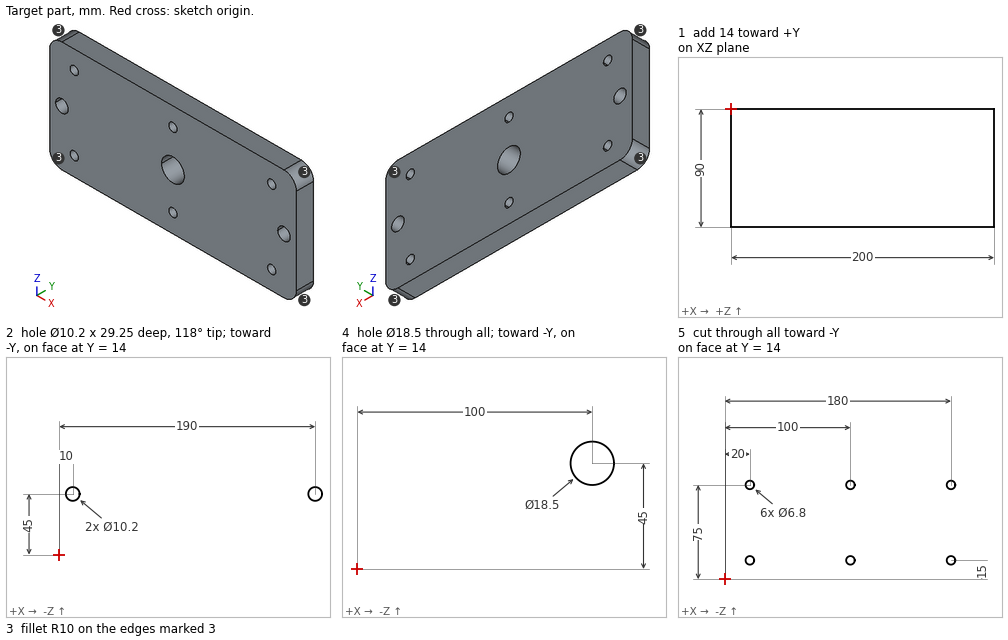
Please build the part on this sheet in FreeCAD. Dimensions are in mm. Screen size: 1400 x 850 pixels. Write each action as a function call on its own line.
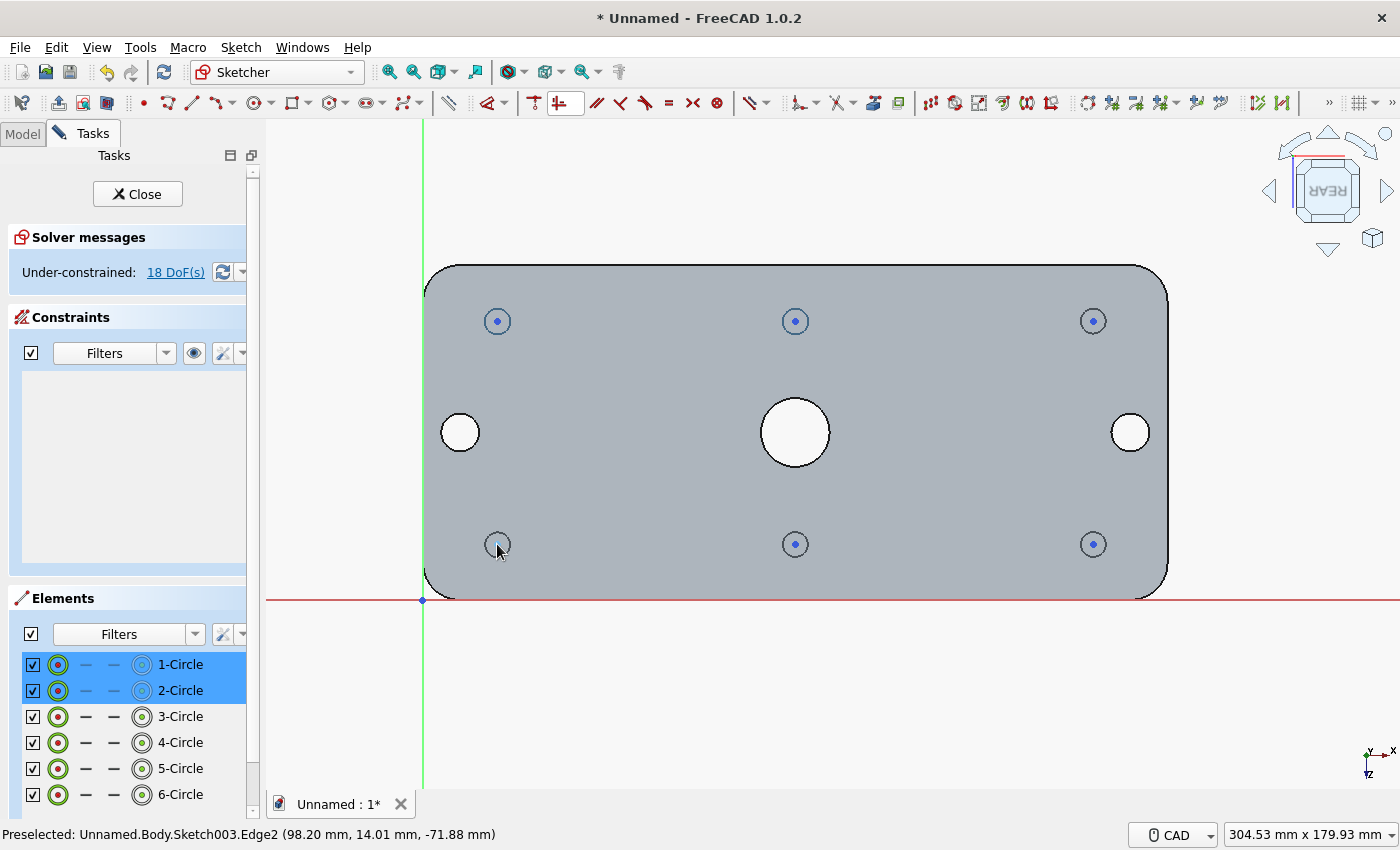
click(1102, 312)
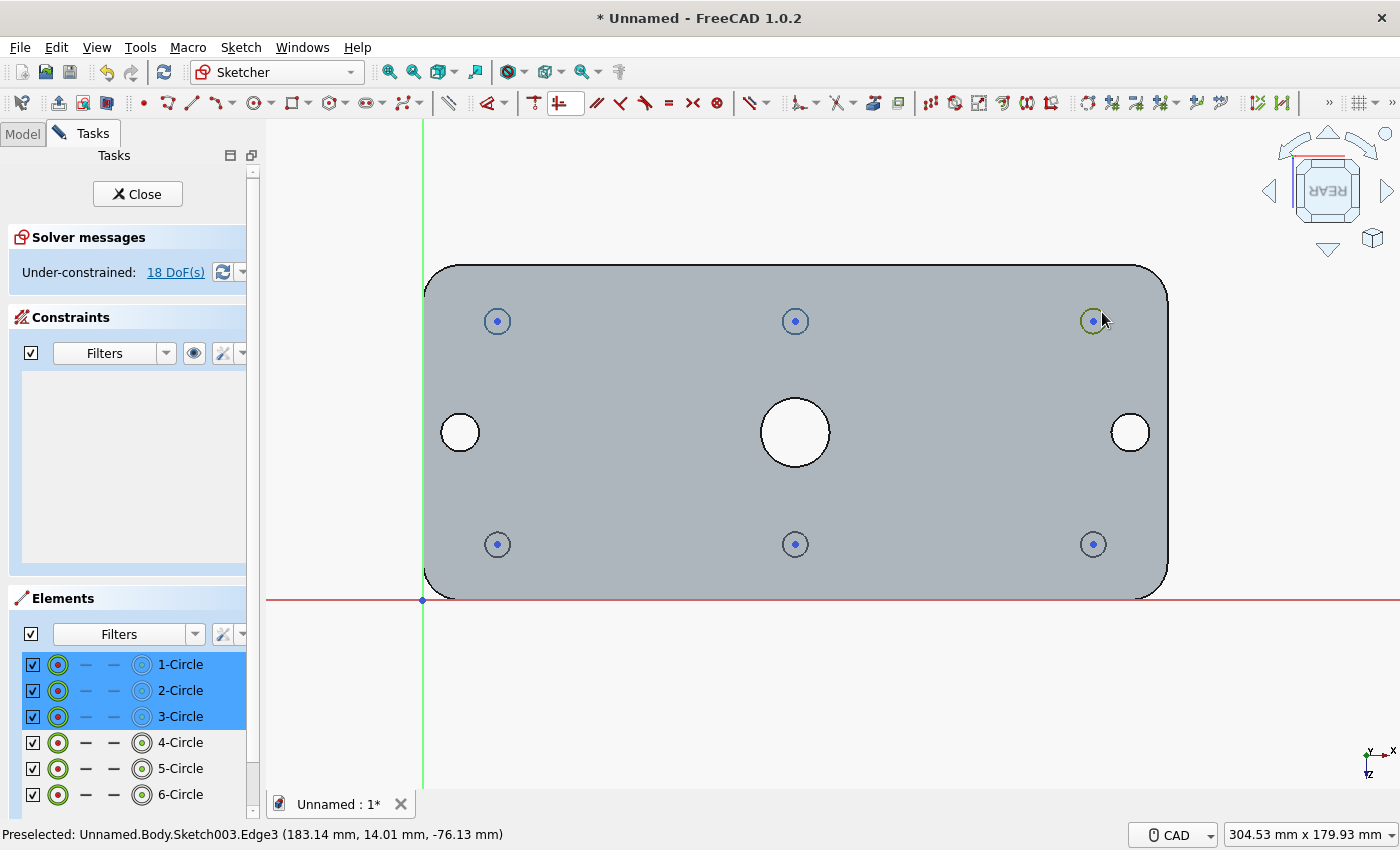
click(1102, 536)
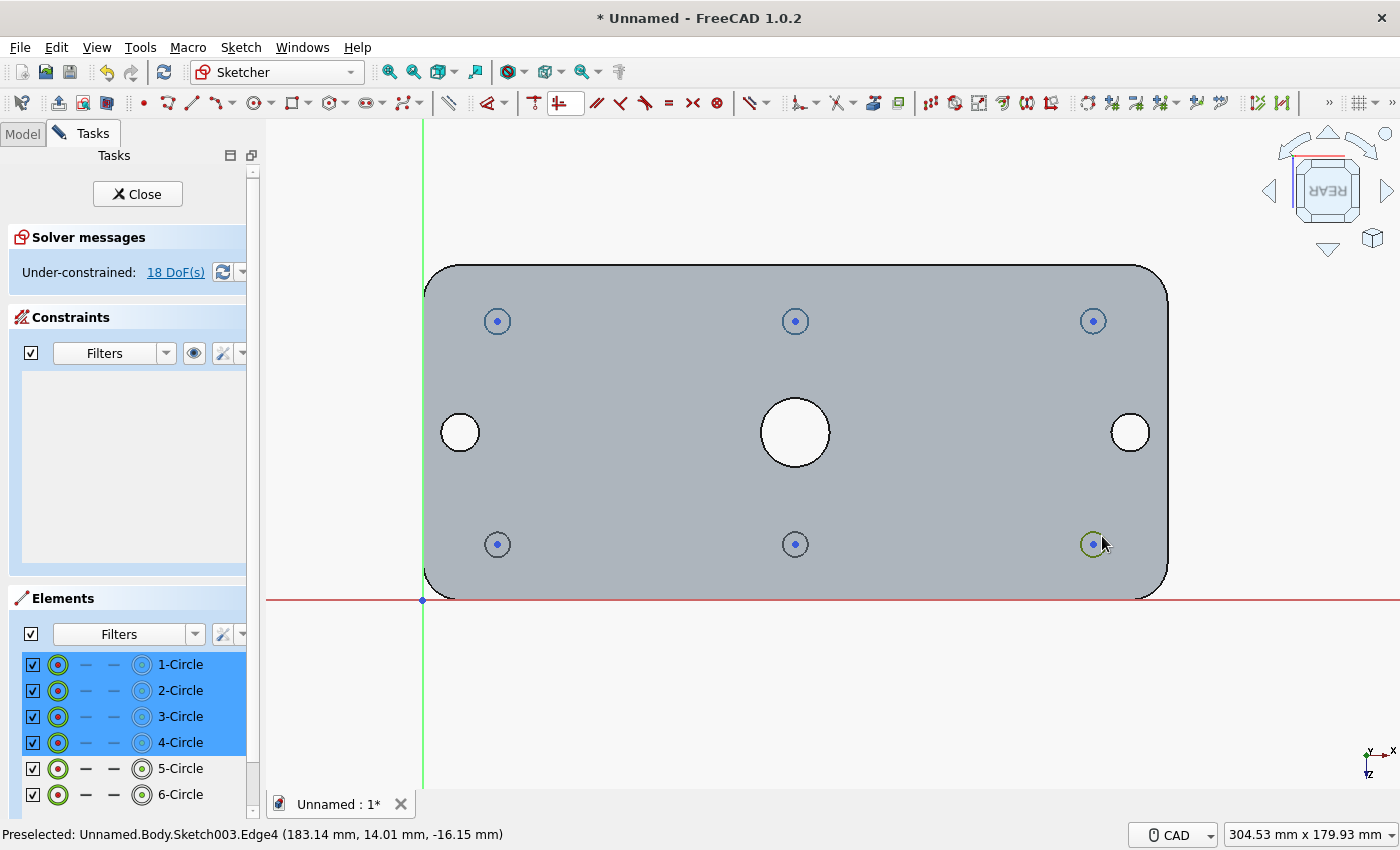
click(804, 536)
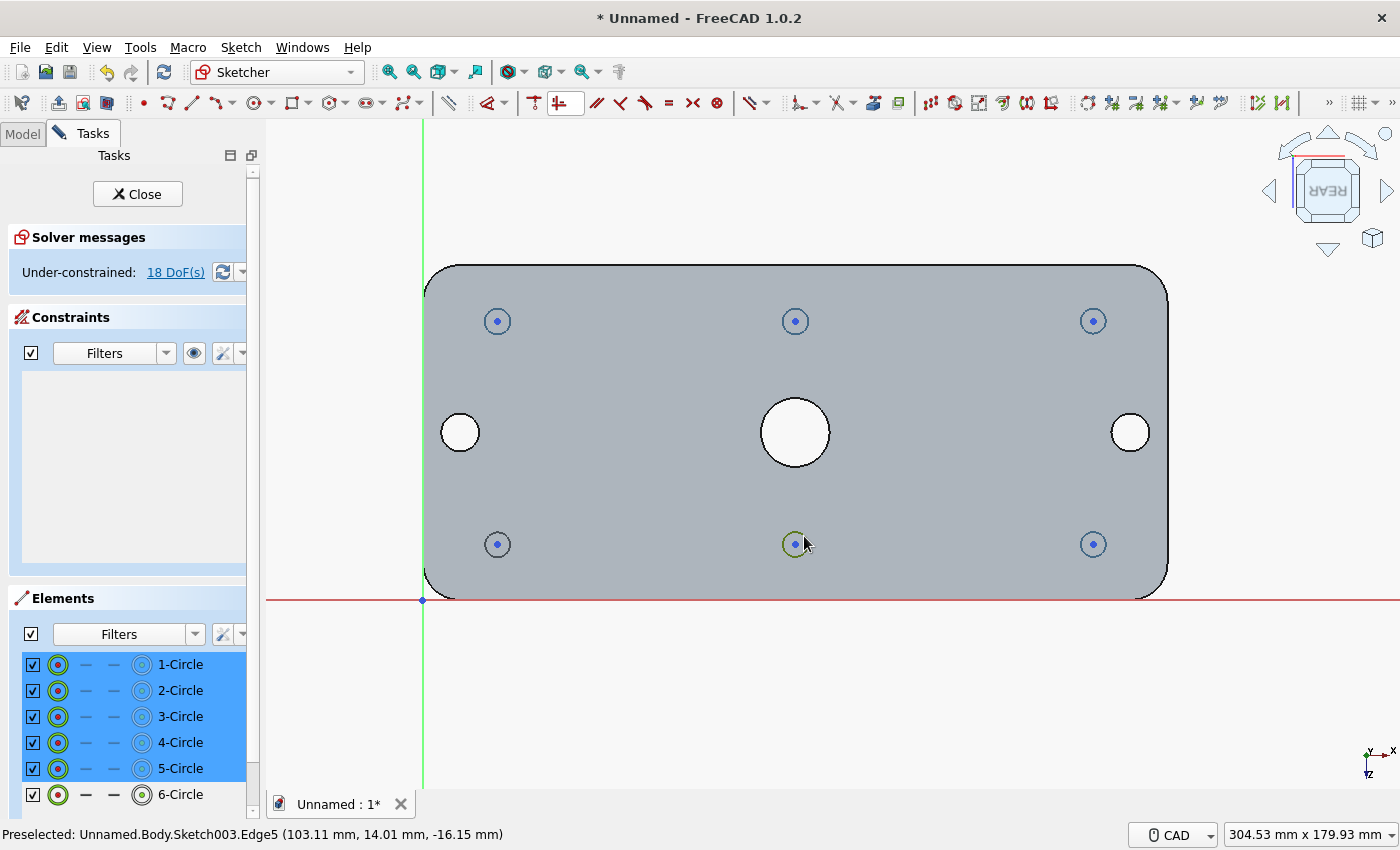
click(506, 536)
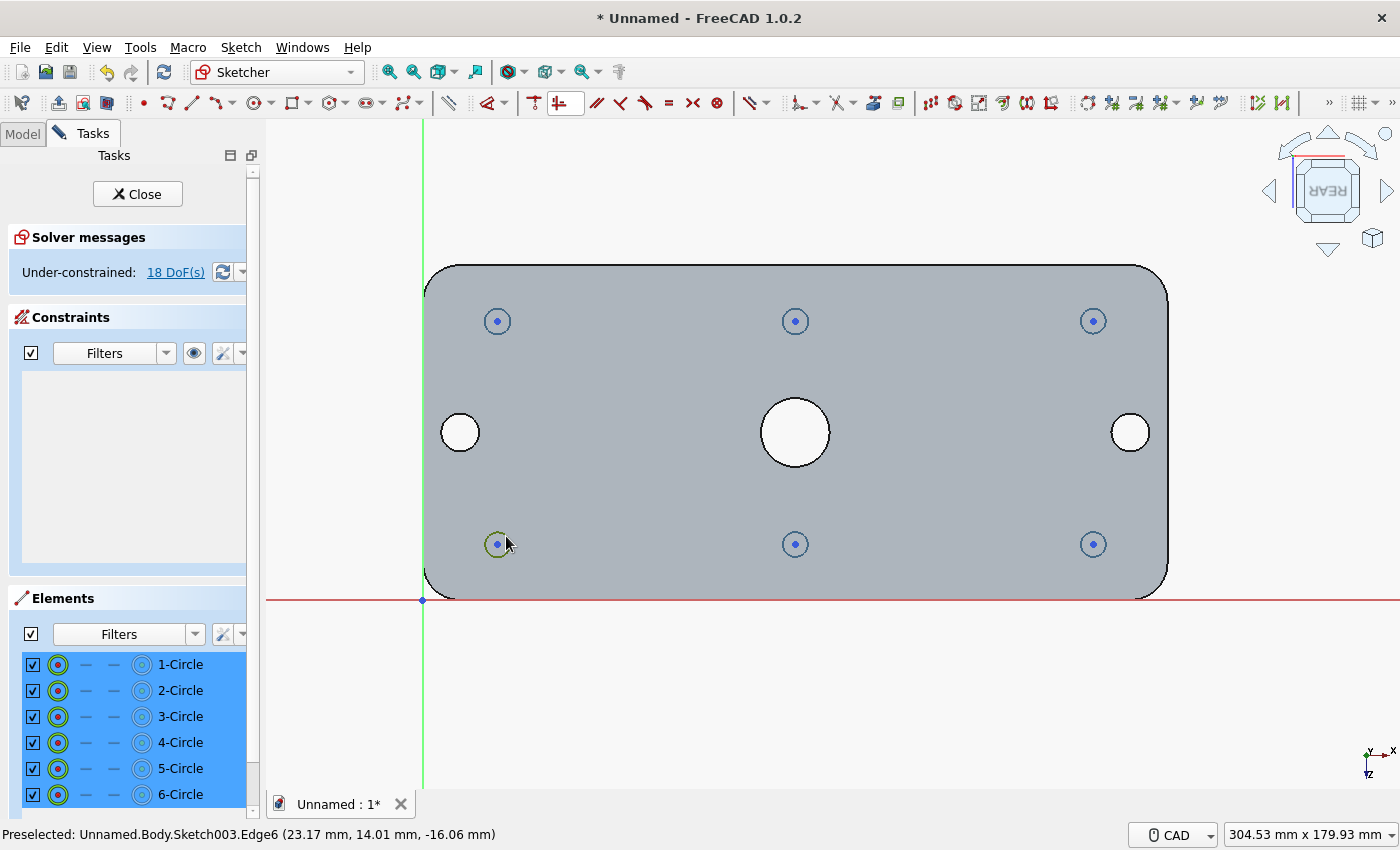
click(670, 104)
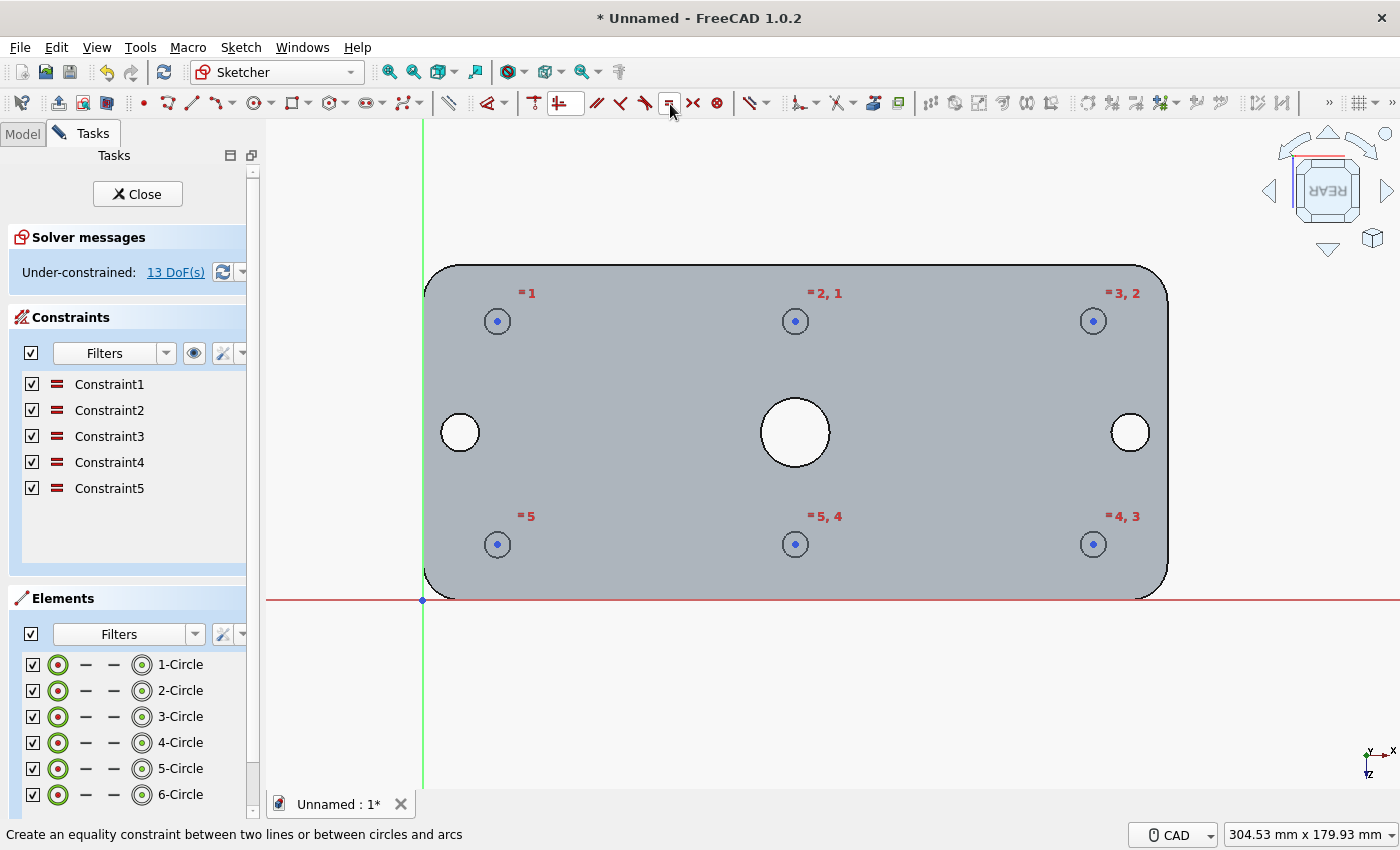
click(497, 322)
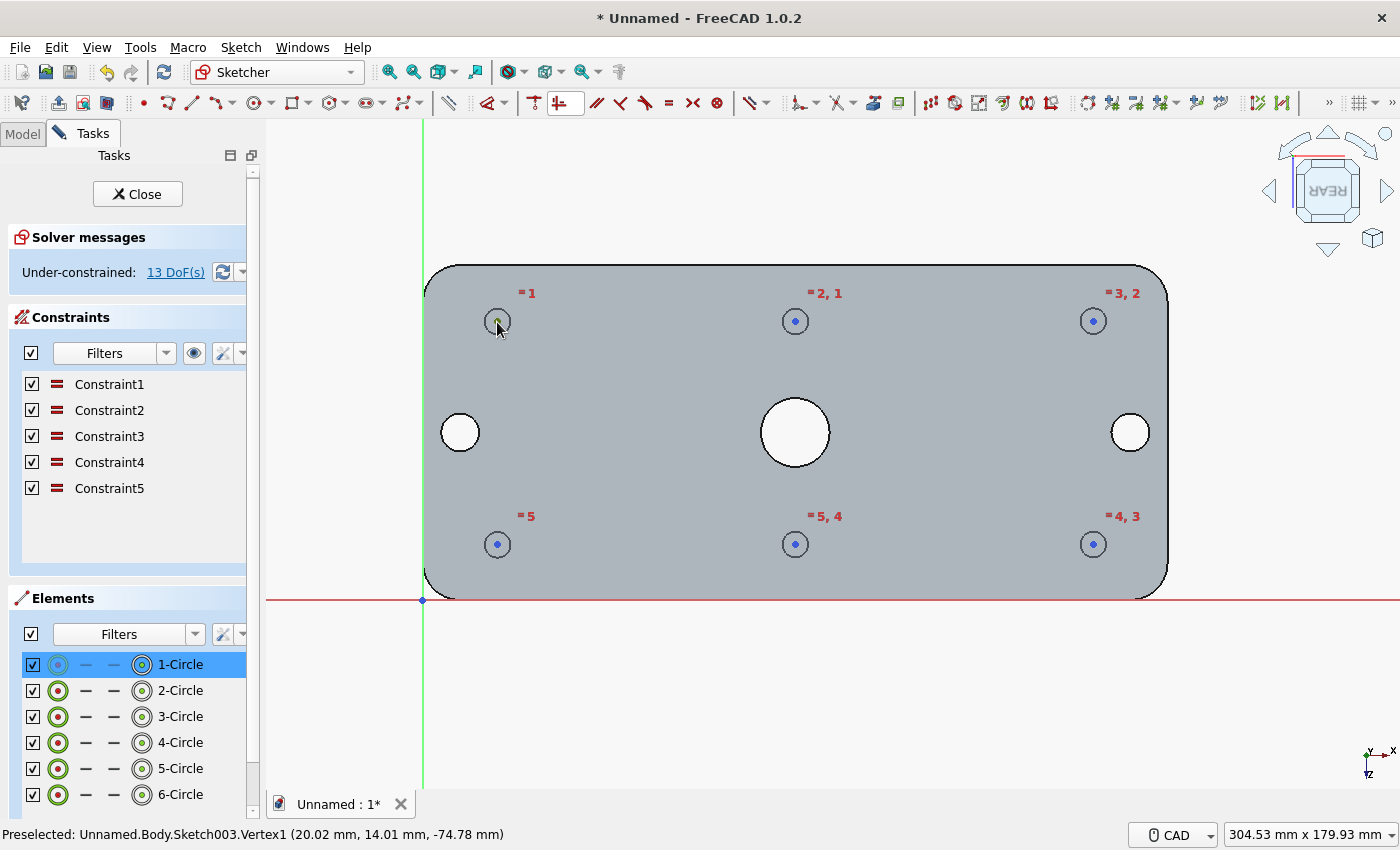
click(795, 322)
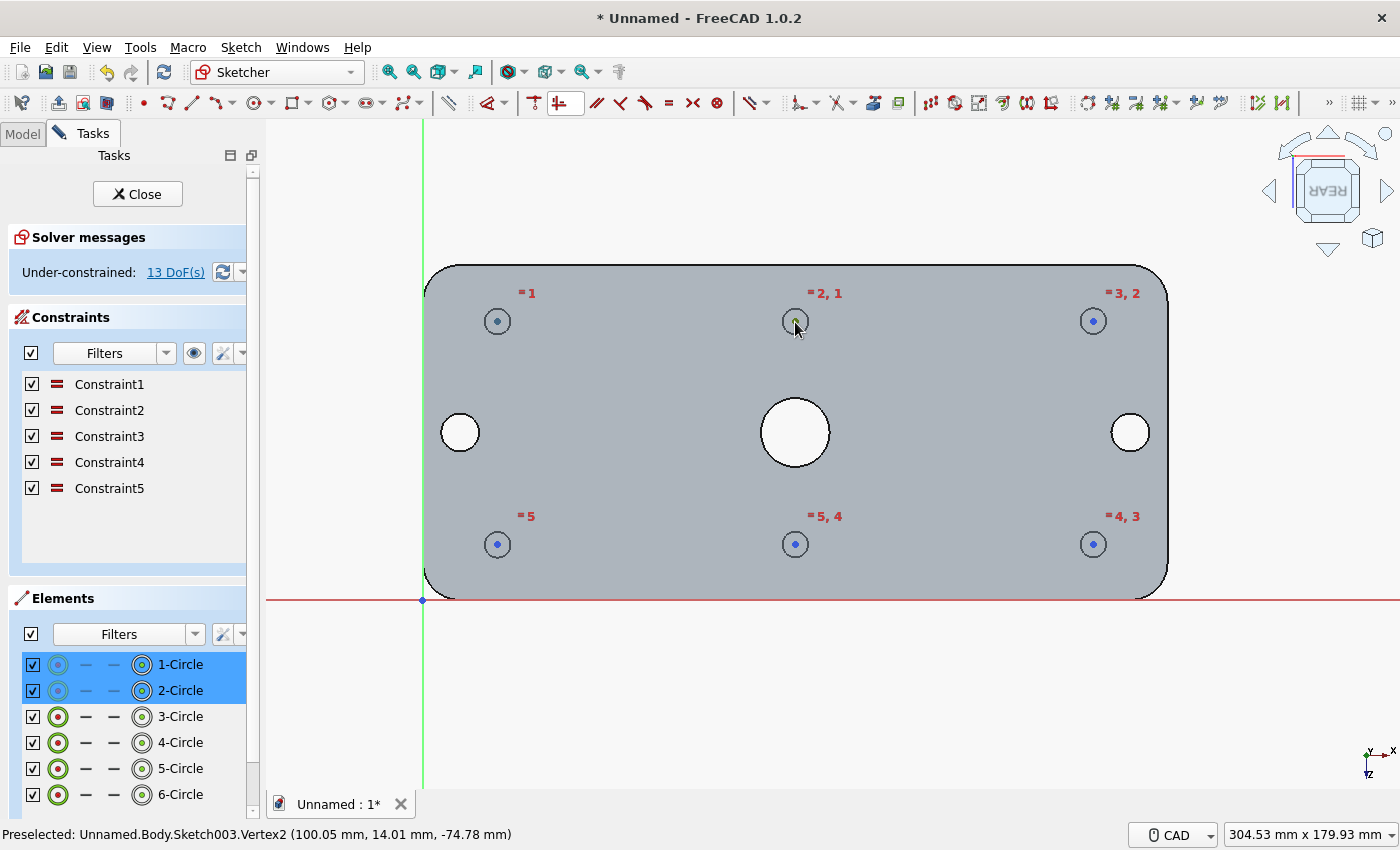
key(h)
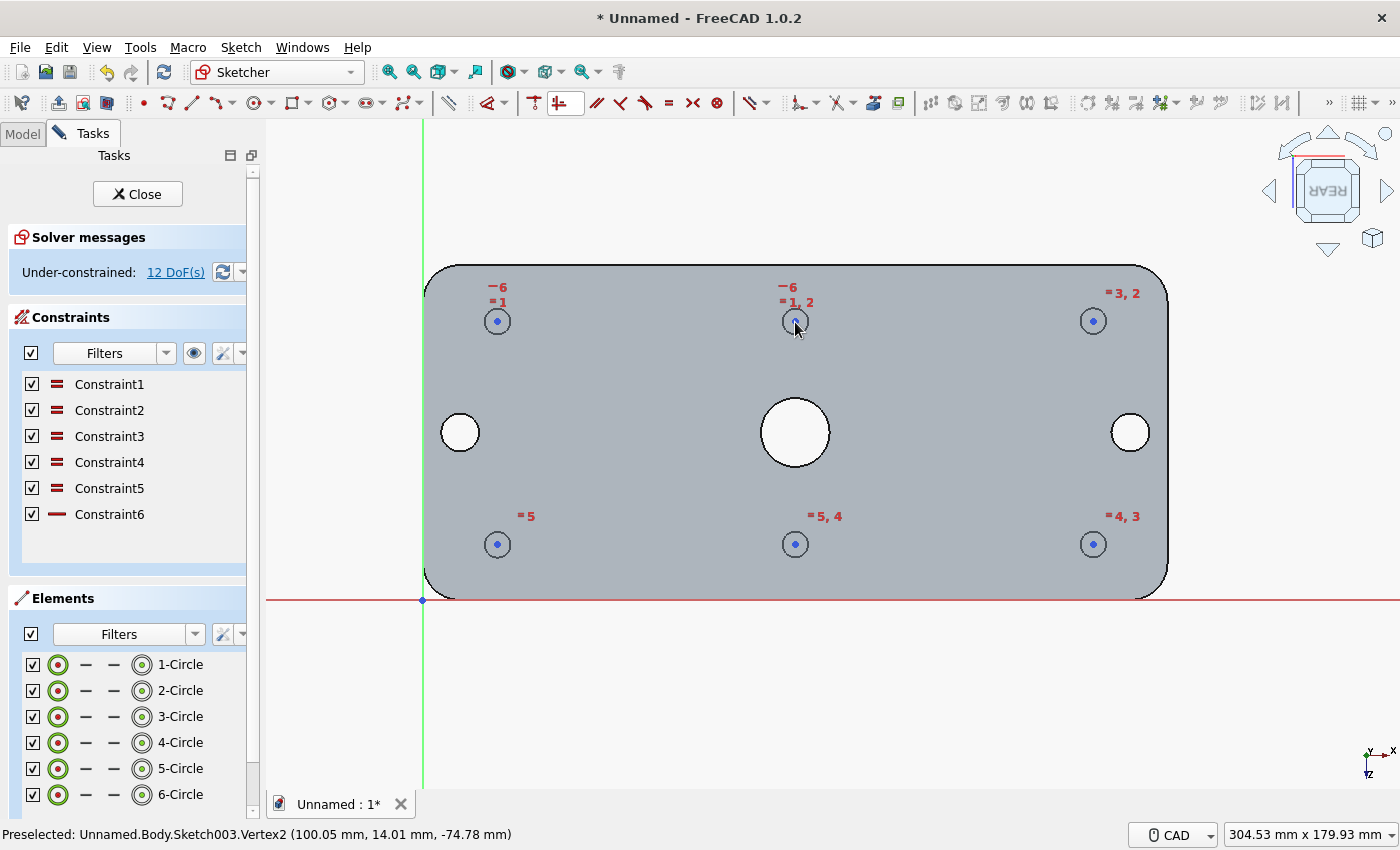
click(795, 322)